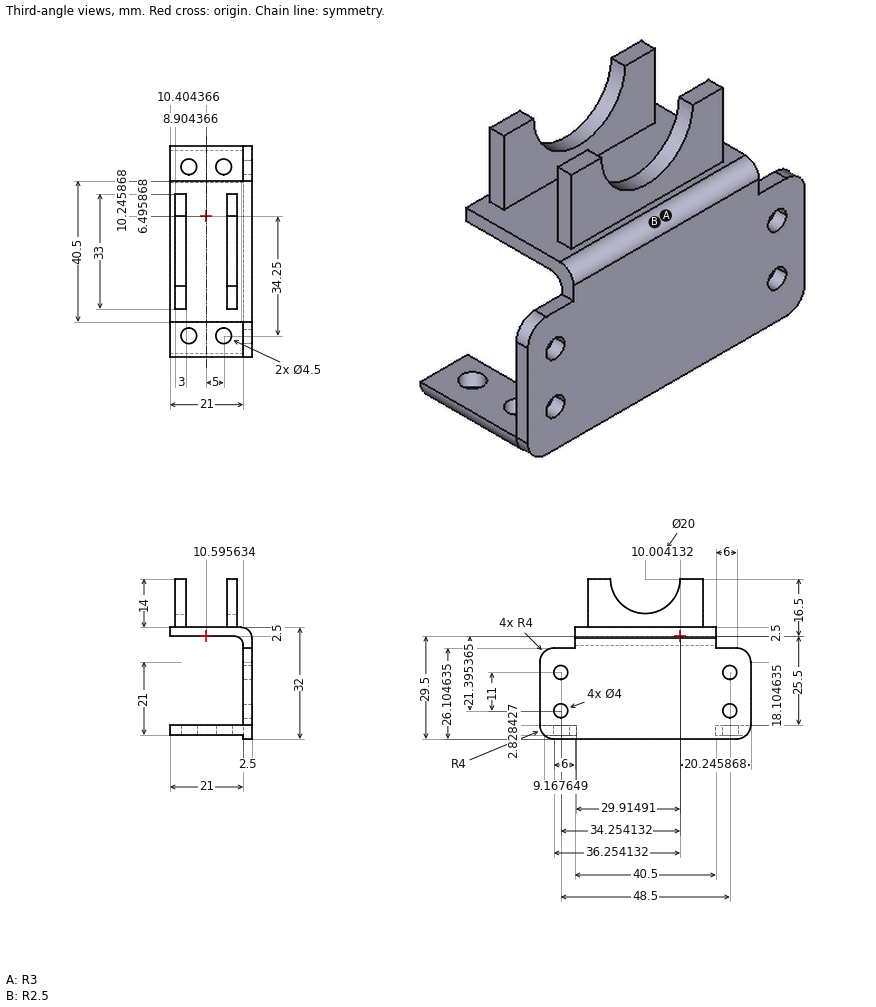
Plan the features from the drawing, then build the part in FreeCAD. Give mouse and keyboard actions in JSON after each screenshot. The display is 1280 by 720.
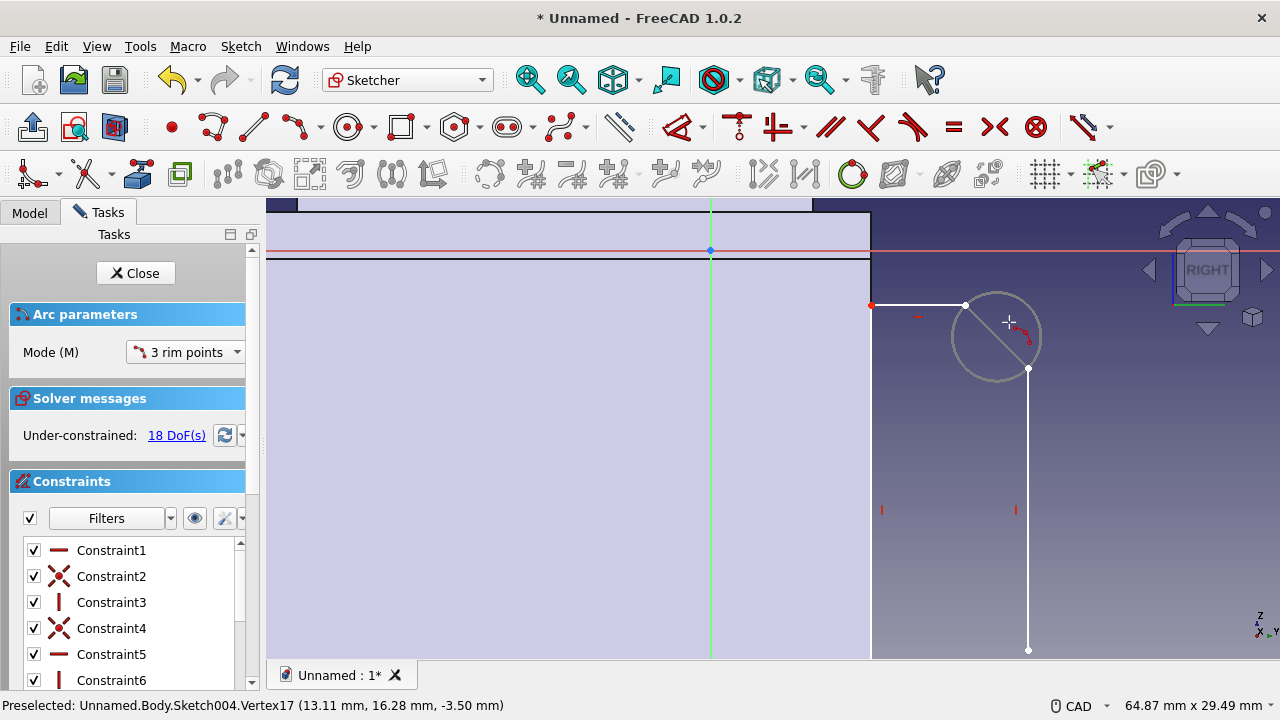
{"action": "left_click", "coordinate": [1009, 322]}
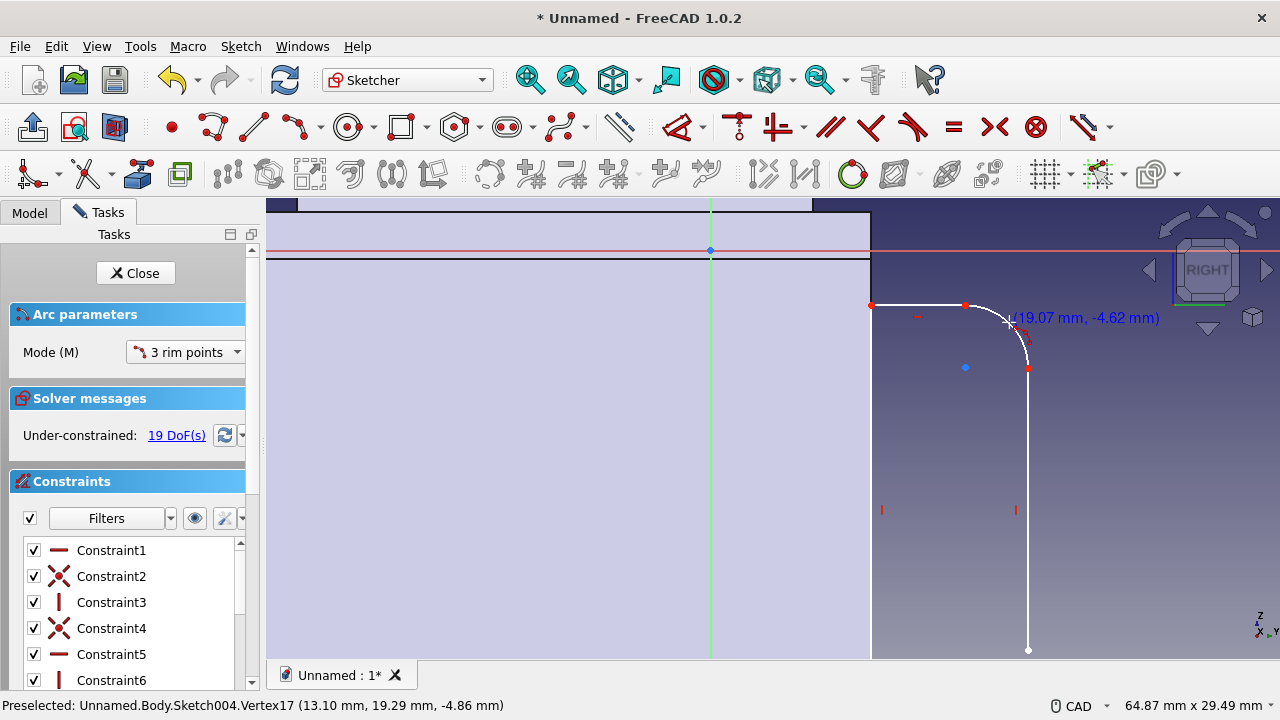
{"action": "scroll", "coordinate": [1009, 321], "scroll_direction": "down", "scroll_amount": 2}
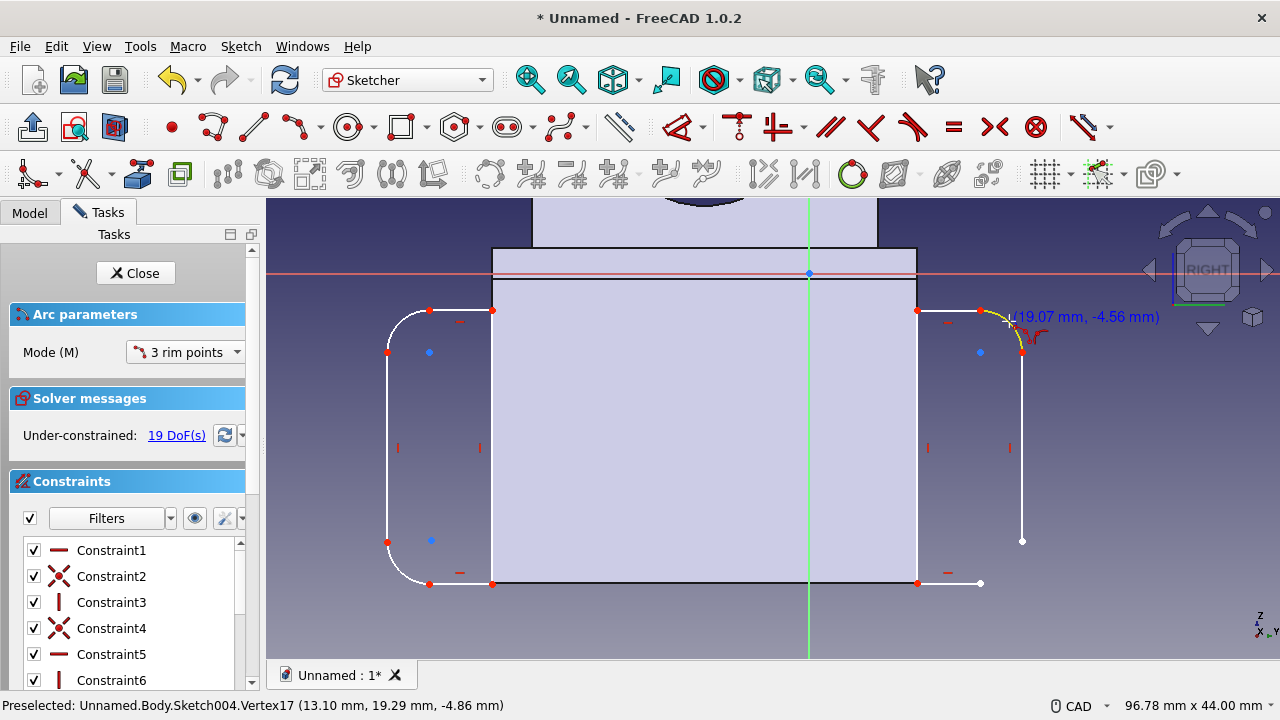
{"action": "left_click", "coordinate": [980, 584]}
{"action": "left_click", "coordinate": [1022, 542]}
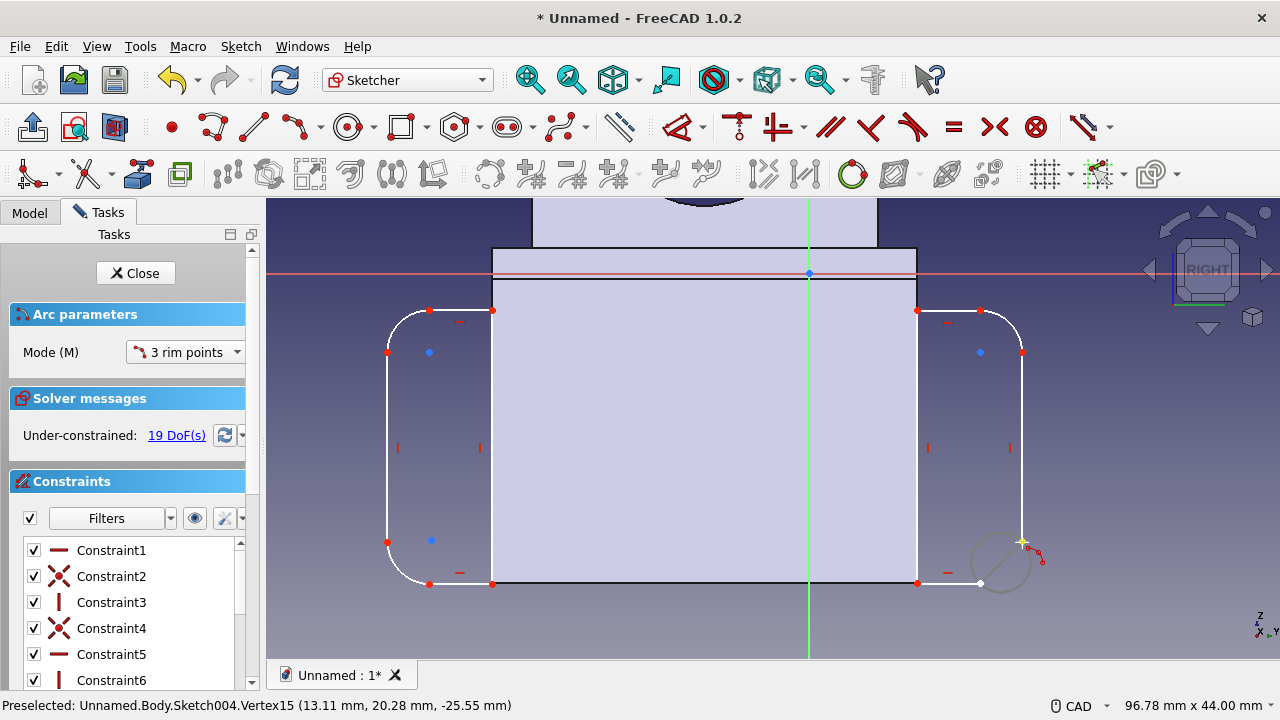
{"action": "scroll", "coordinate": [1009, 571], "scroll_direction": "up", "scroll_amount": 2}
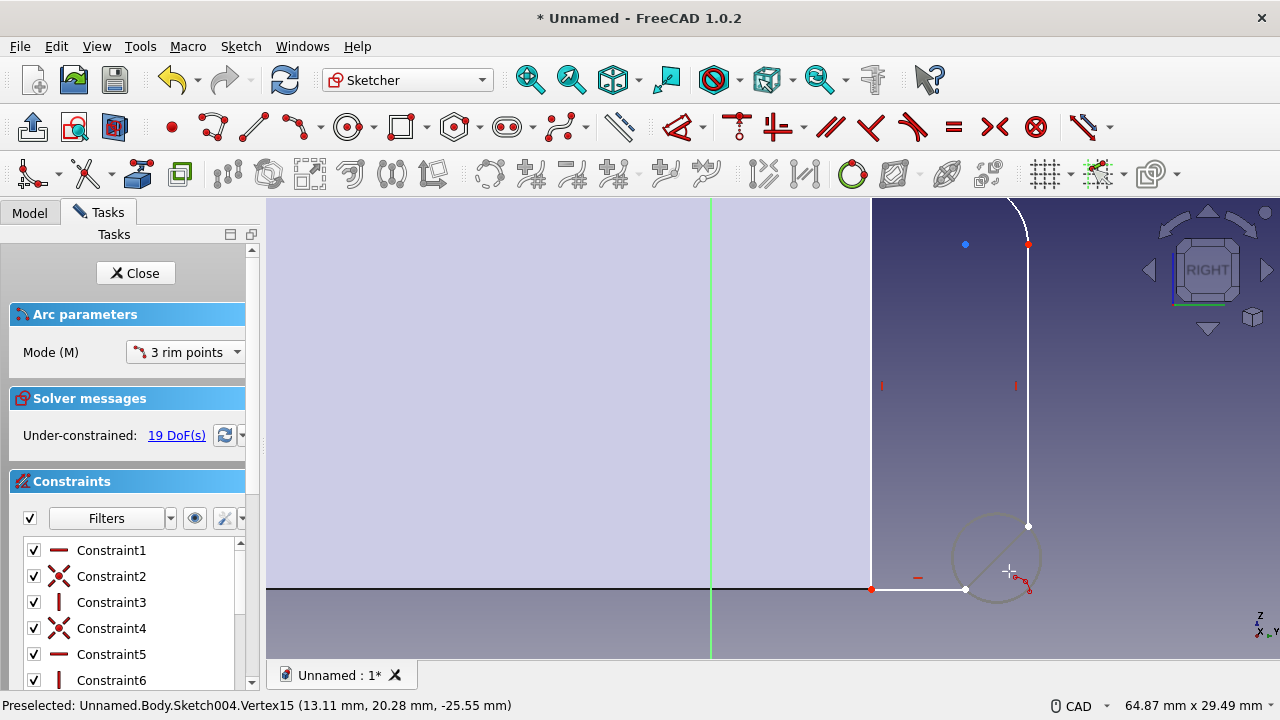
{"action": "left_click", "coordinate": [1009, 570]}
{"action": "key", "text": "Escape"}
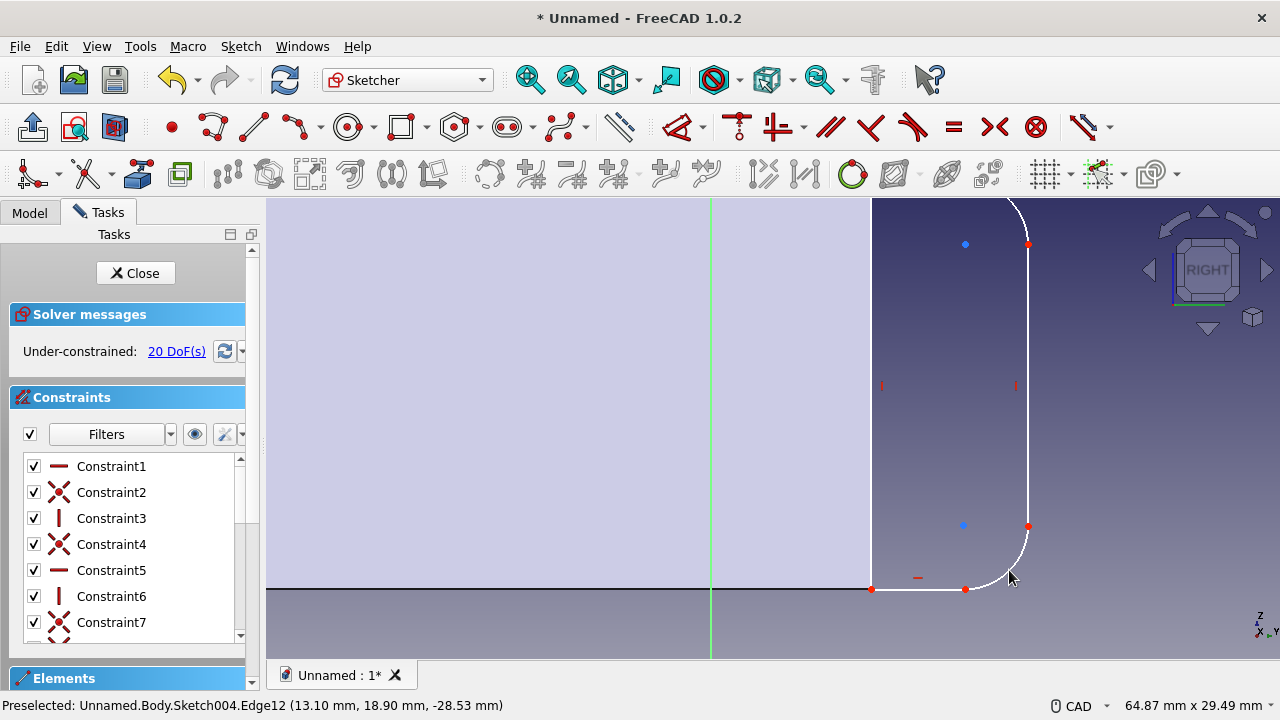
{"action": "scroll", "coordinate": [1009, 572], "scroll_direction": "down", "scroll_amount": 2}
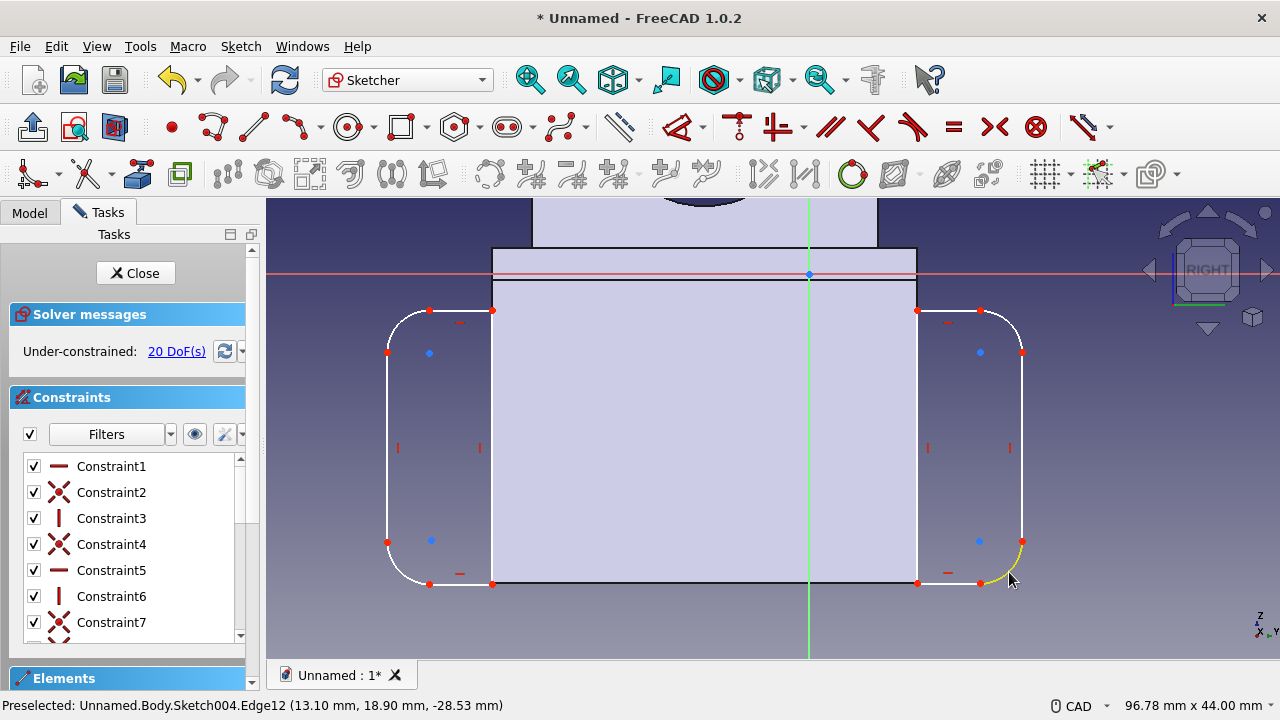
{"action": "left_click", "coordinate": [448, 585]}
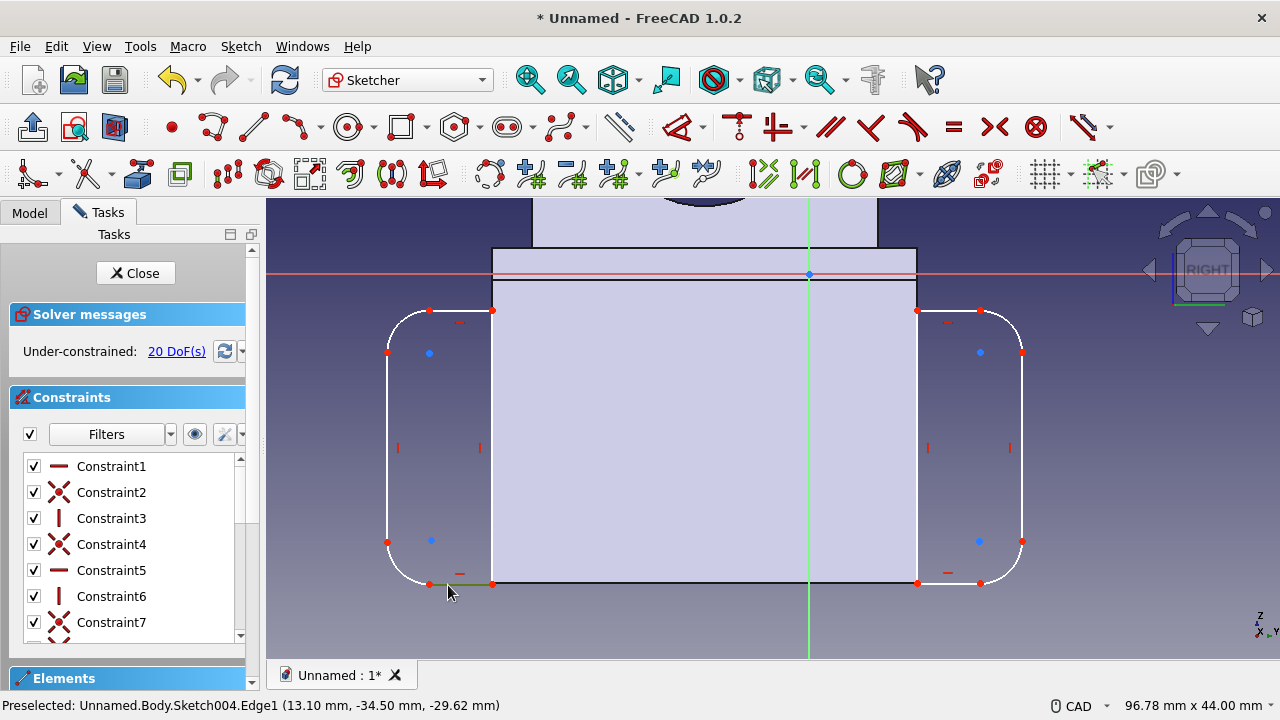
{"action": "left_click", "coordinate": [392, 561]}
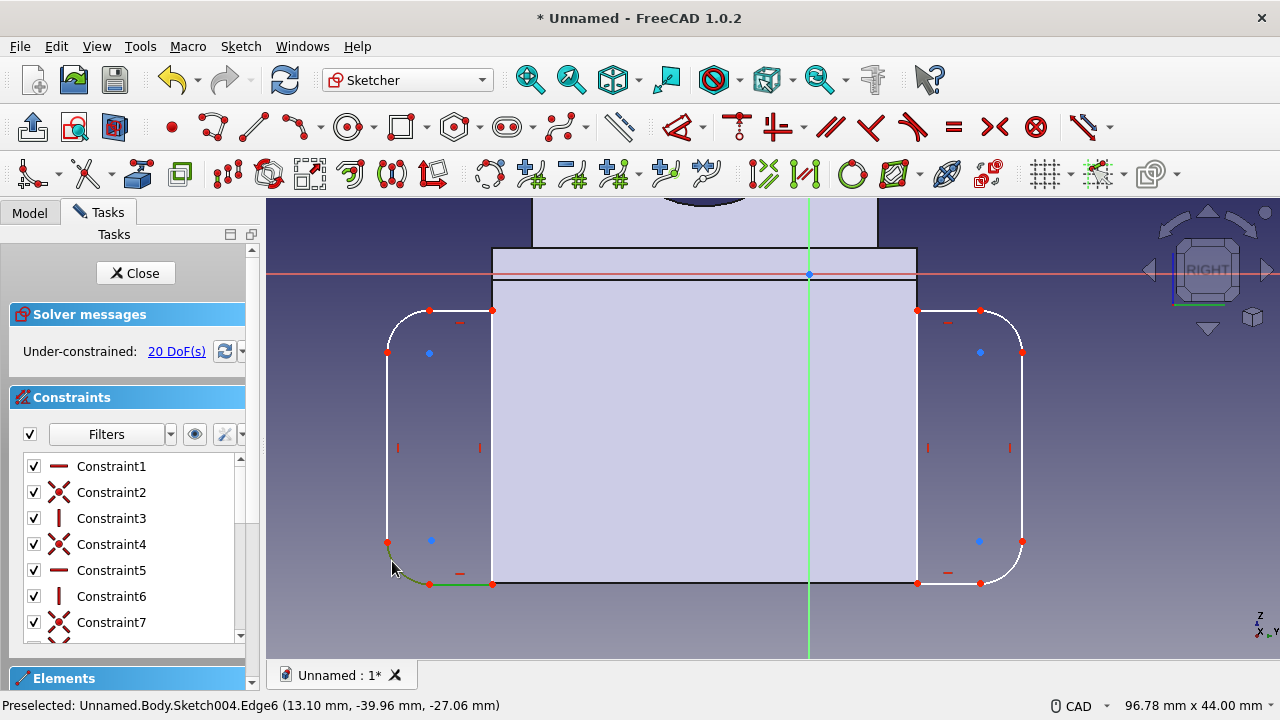
{"action": "left_click", "coordinate": [913, 128]}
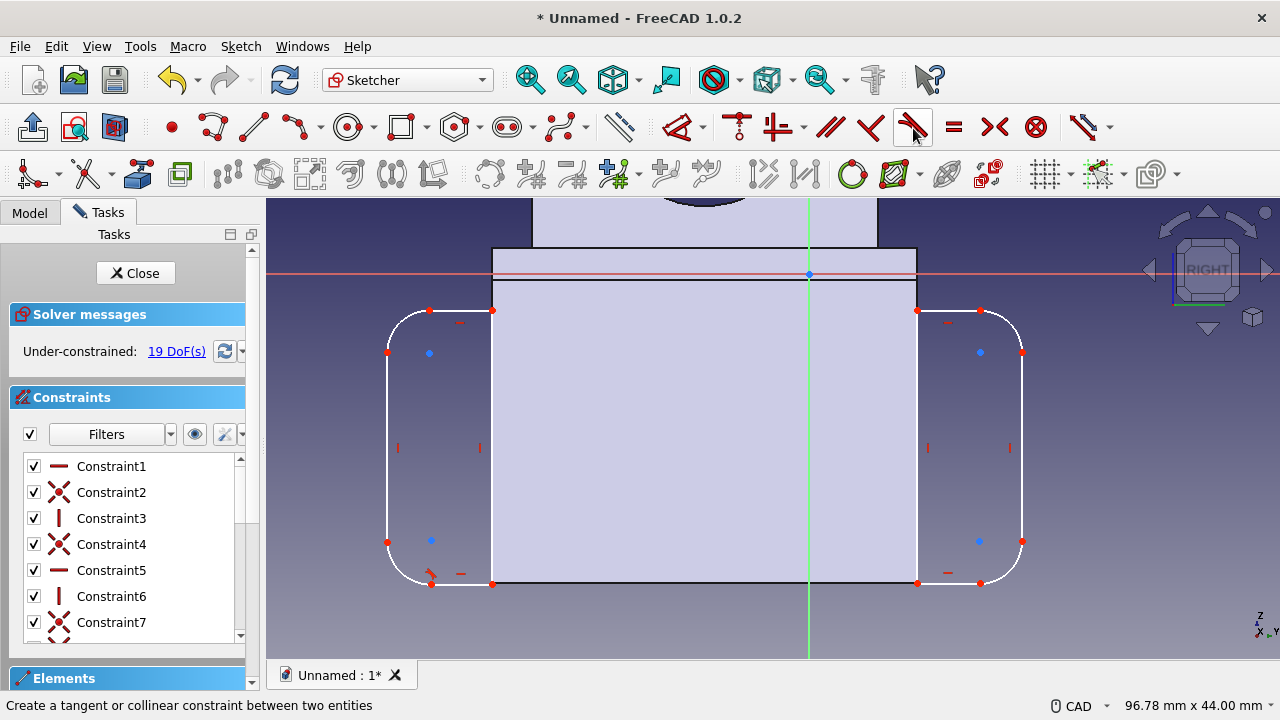
{"action": "left_click", "coordinate": [473, 311]}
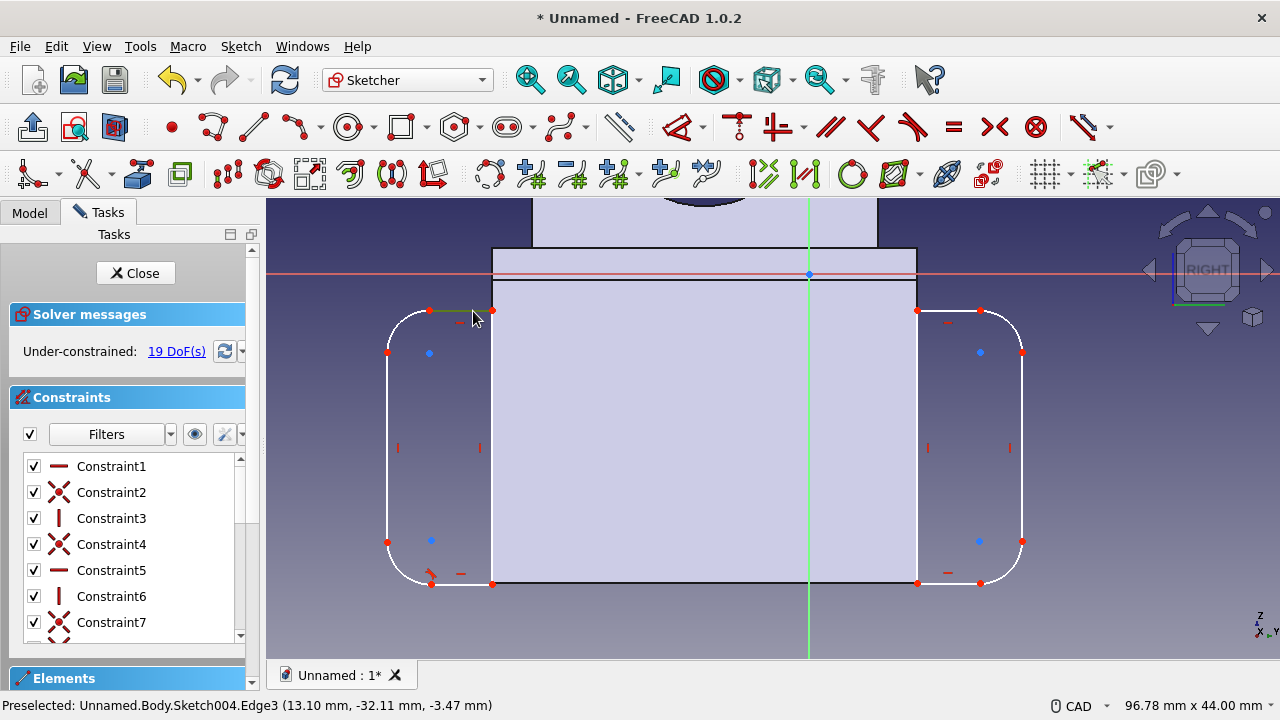
{"action": "left_click", "coordinate": [410, 315]}